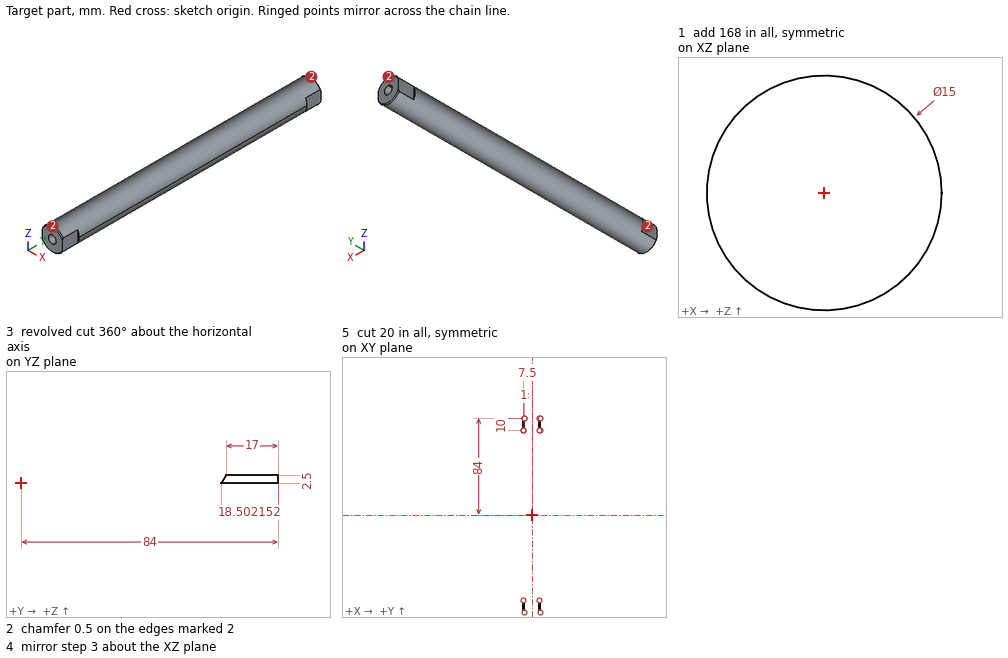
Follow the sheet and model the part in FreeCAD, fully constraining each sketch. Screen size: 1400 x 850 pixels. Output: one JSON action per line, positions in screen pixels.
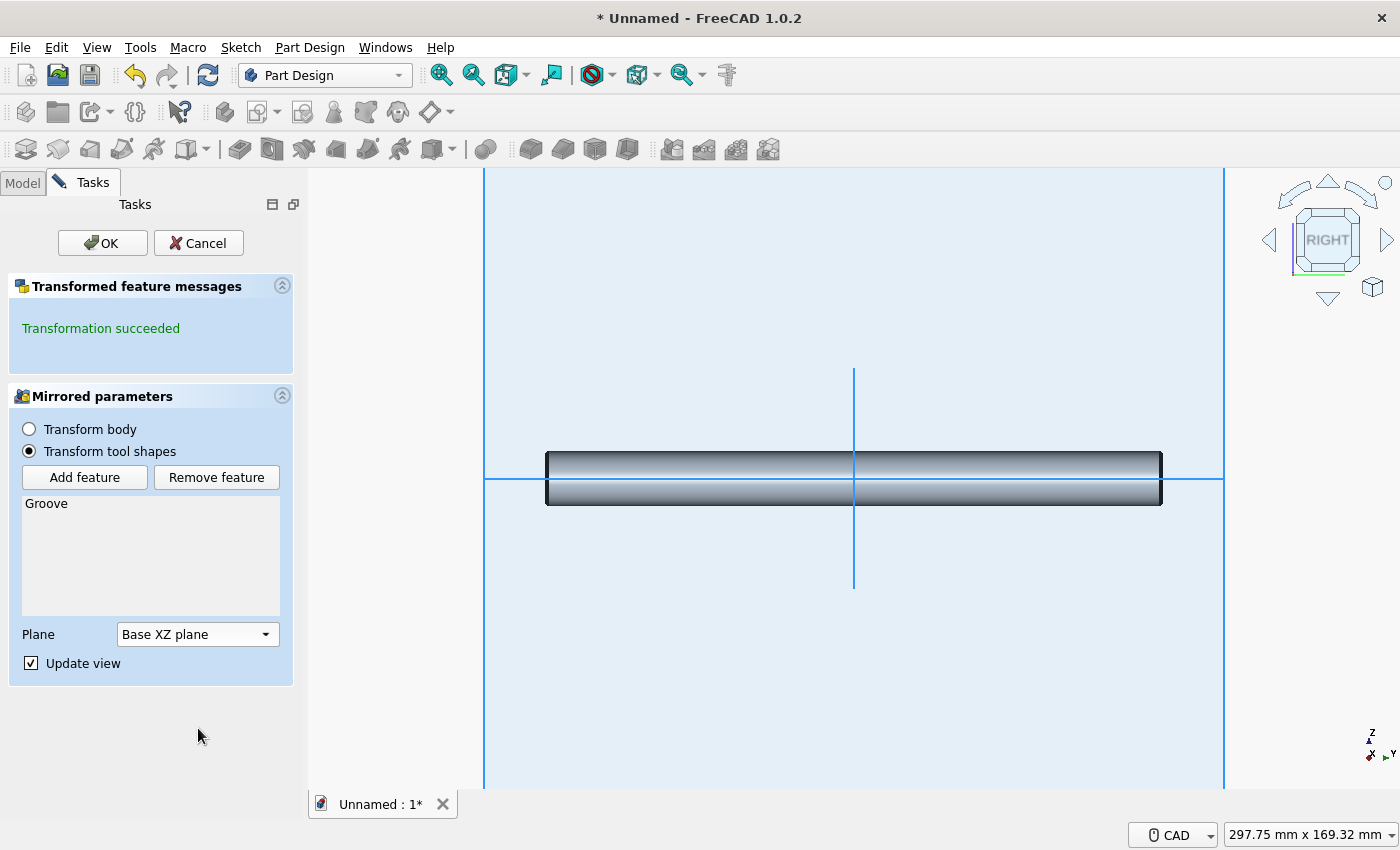
{"action": "left_click", "coordinate": [103, 243]}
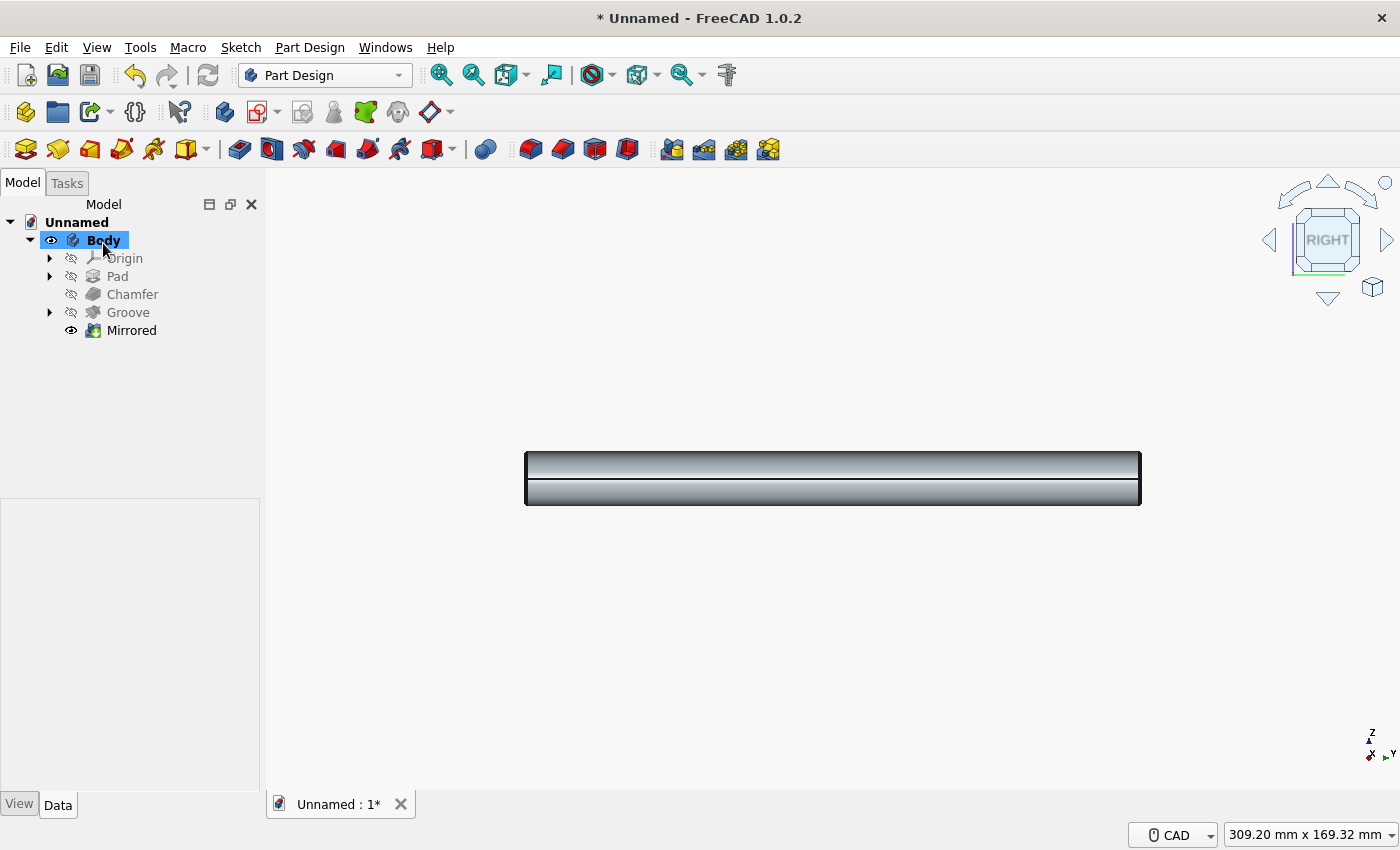
{"action": "left_click", "coordinate": [258, 112]}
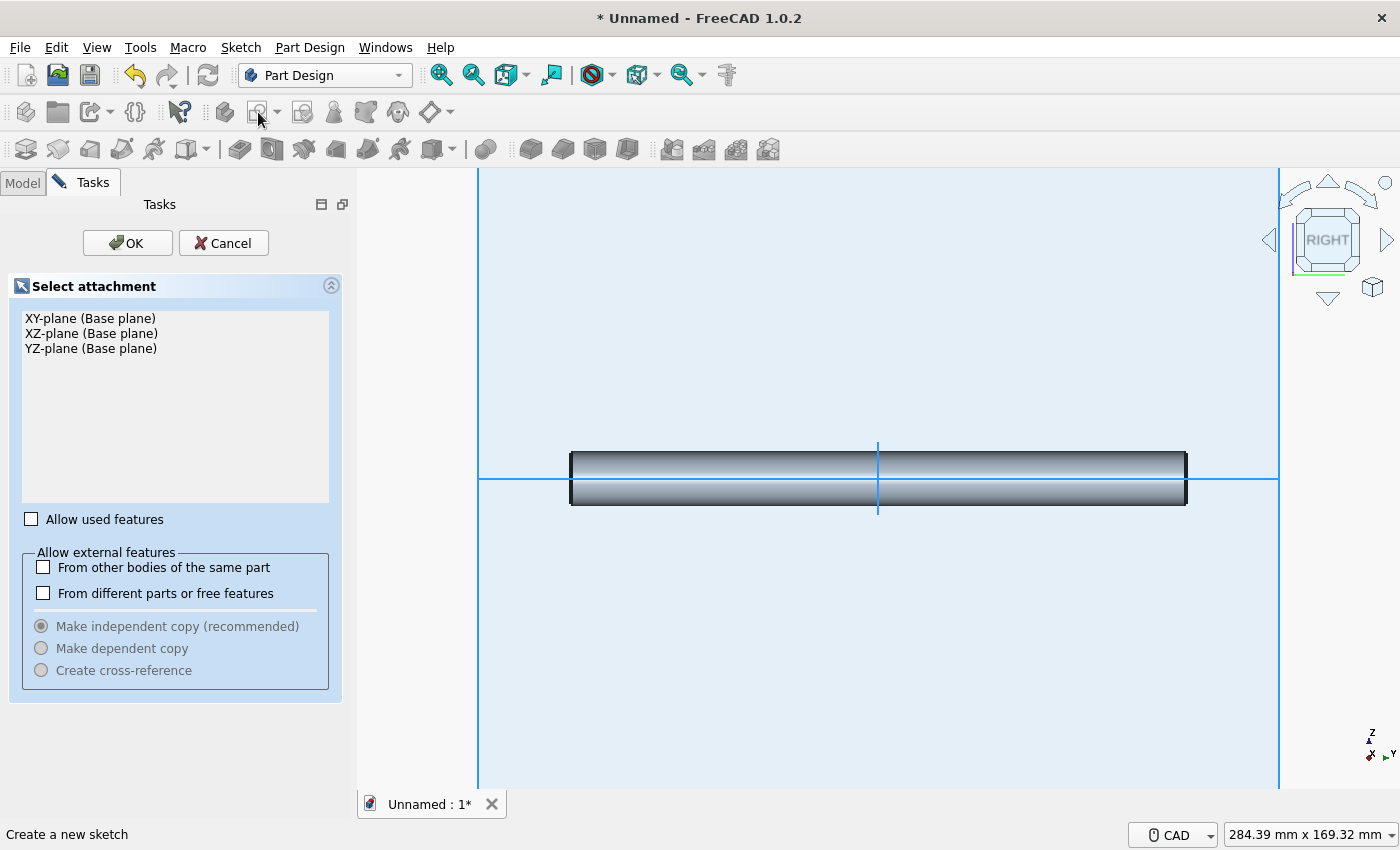
{"action": "left_click", "coordinate": [82, 318]}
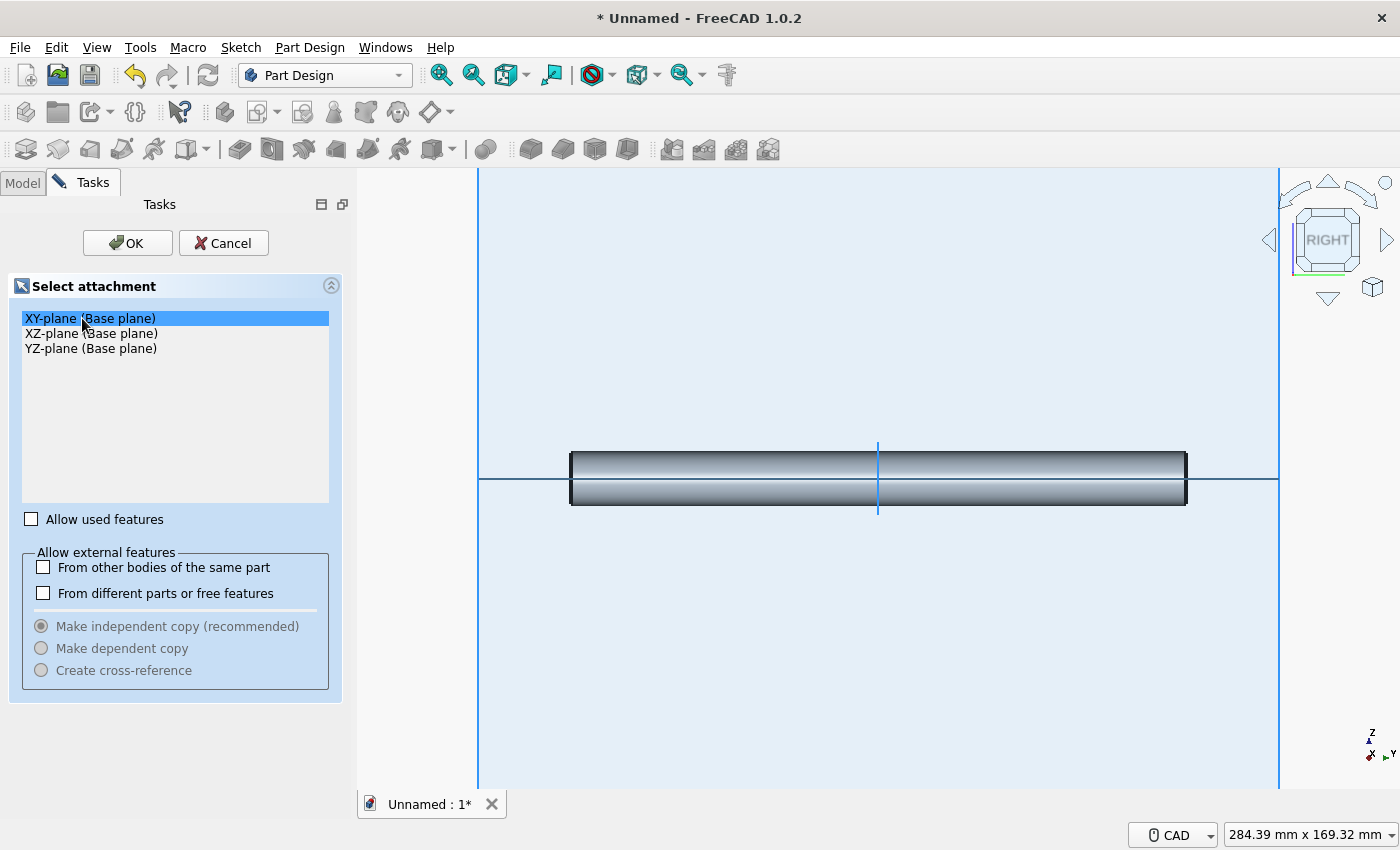
{"action": "left_click", "coordinate": [128, 243]}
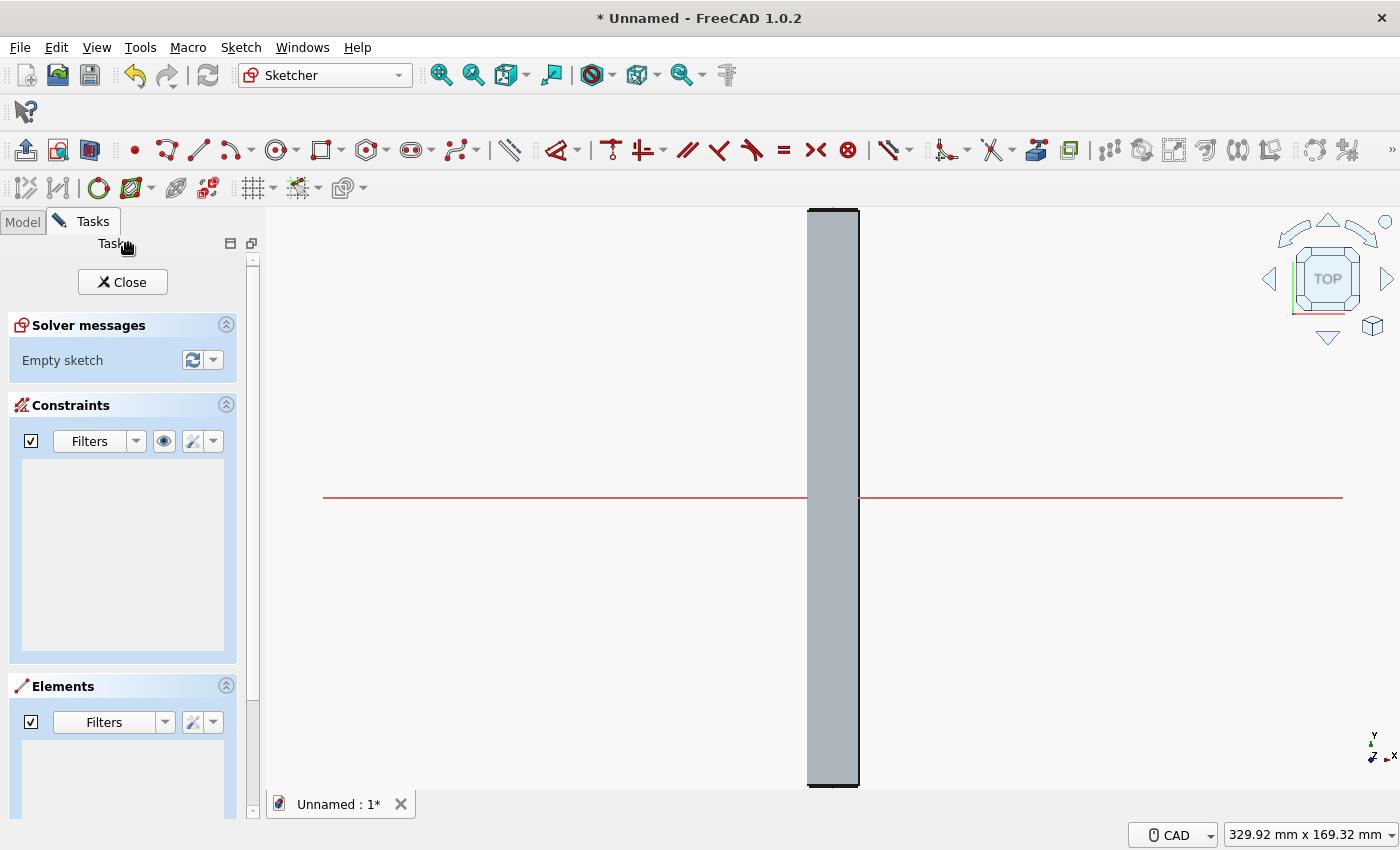
{"action": "left_click", "coordinate": [90, 150]}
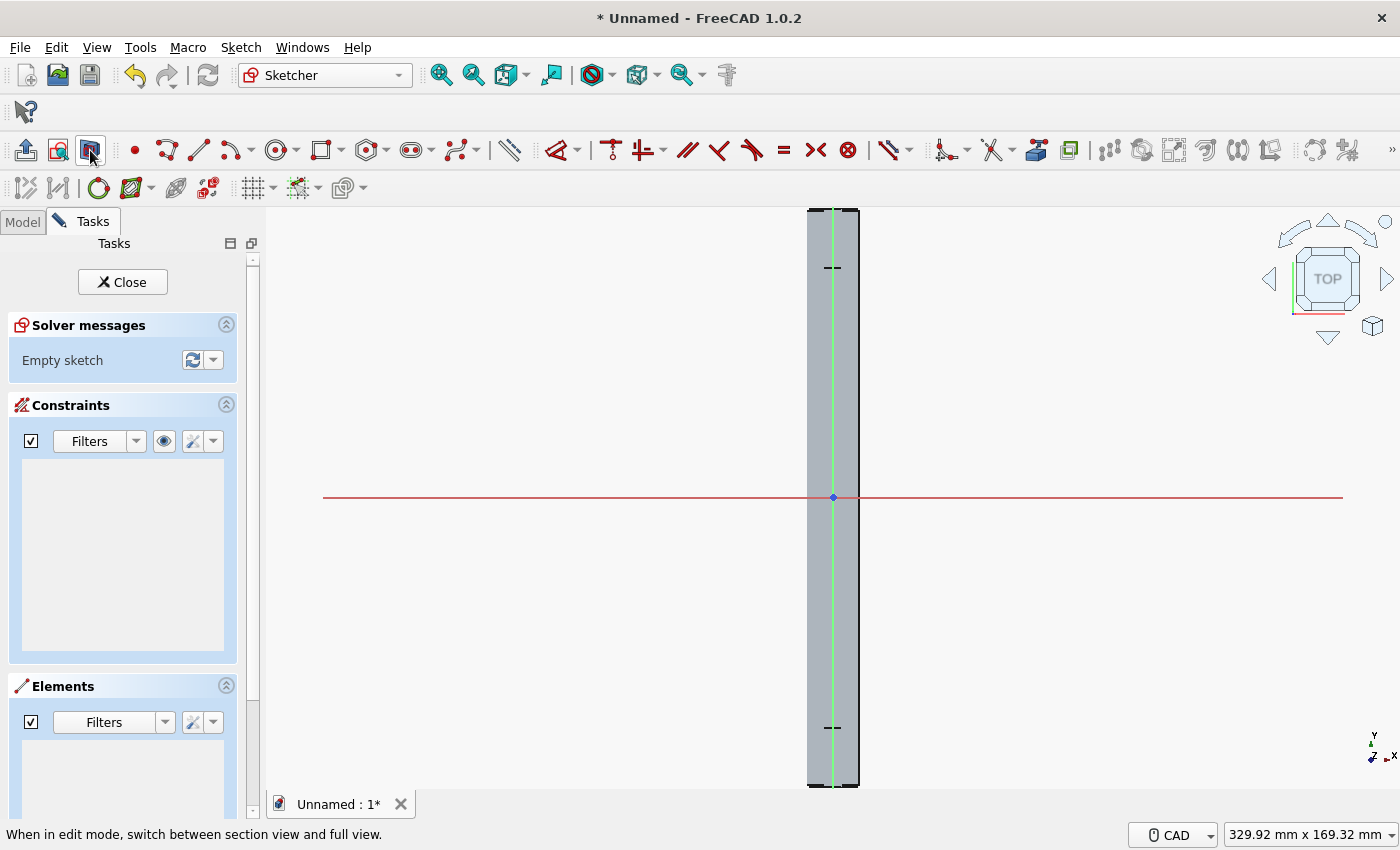
{"action": "scroll", "coordinate": [625, 498], "scroll_direction": "down", "scroll_amount": 2}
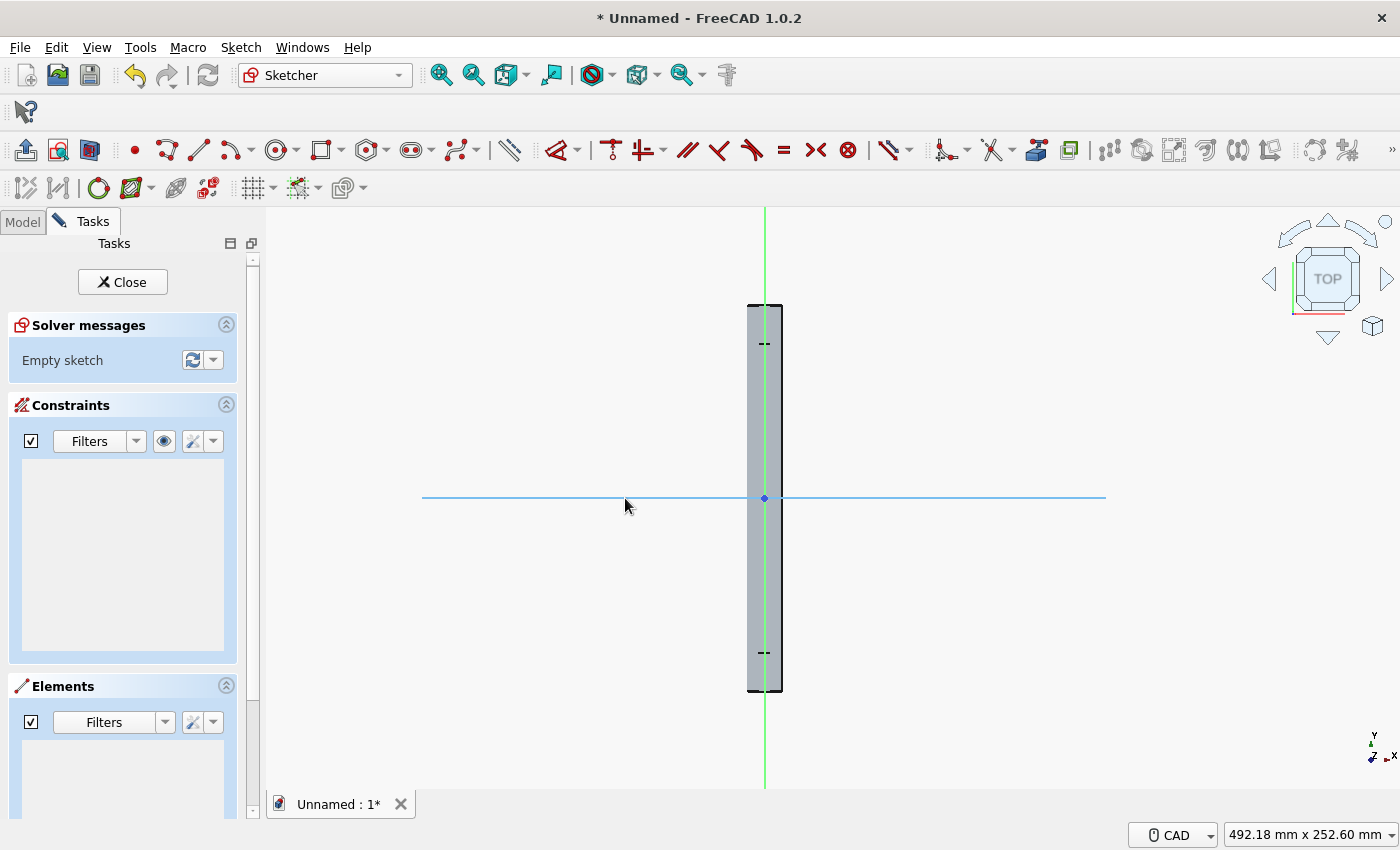
{"action": "left_click", "coordinate": [322, 150]}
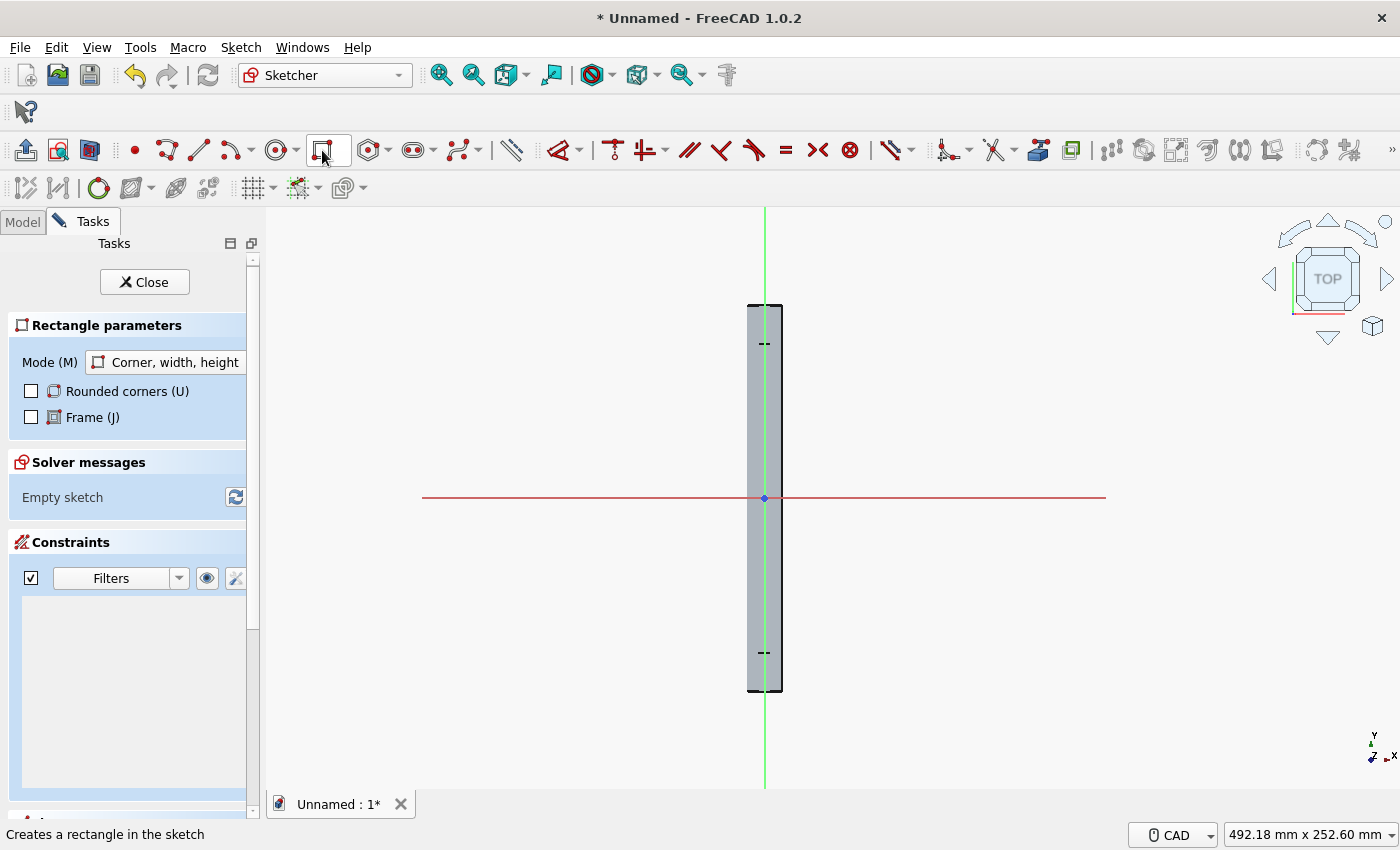
{"action": "scroll", "coordinate": [747, 305], "scroll_direction": "up", "scroll_amount": 10}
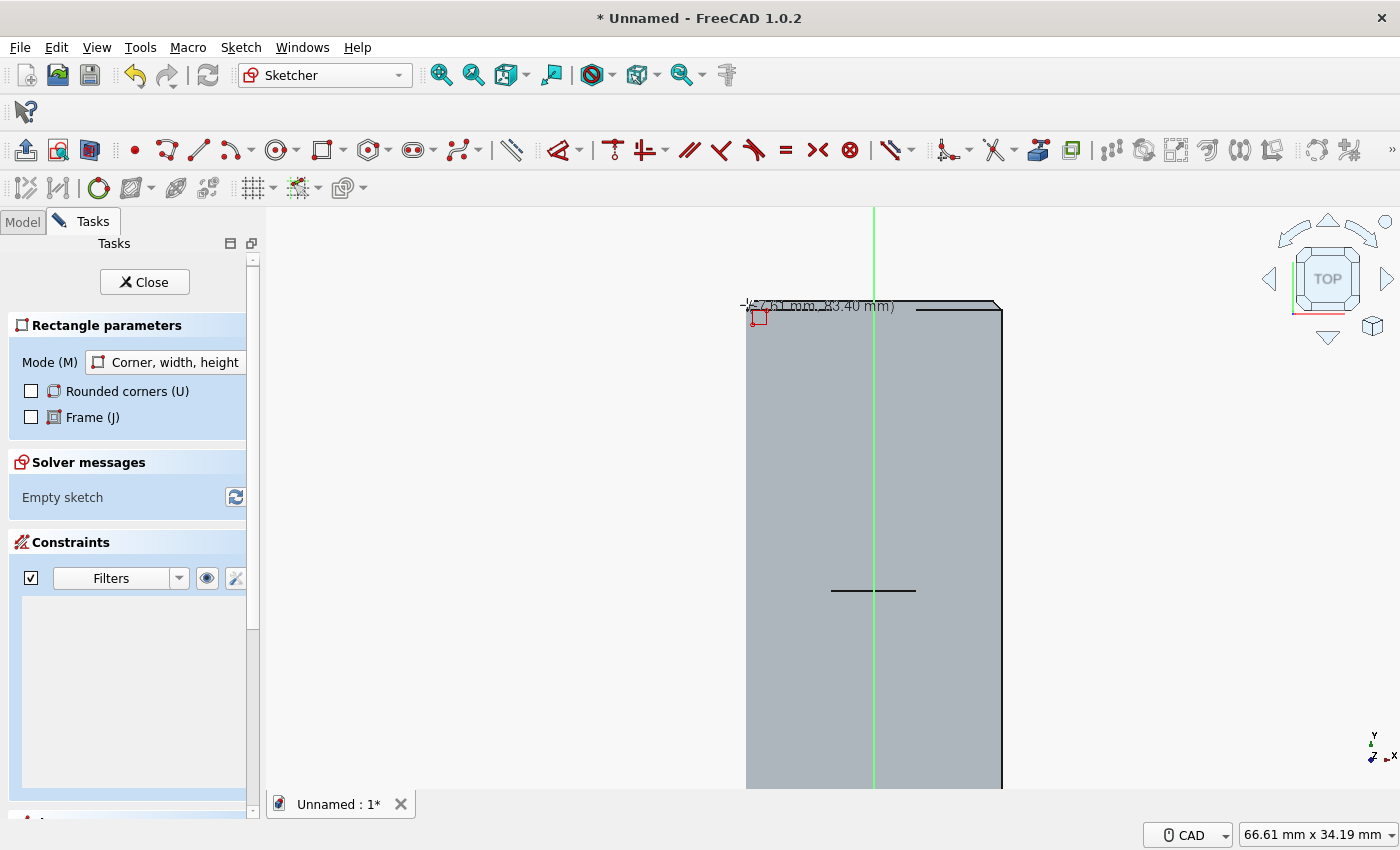
{"action": "scroll", "coordinate": [747, 305], "scroll_direction": "down", "scroll_amount": 10}